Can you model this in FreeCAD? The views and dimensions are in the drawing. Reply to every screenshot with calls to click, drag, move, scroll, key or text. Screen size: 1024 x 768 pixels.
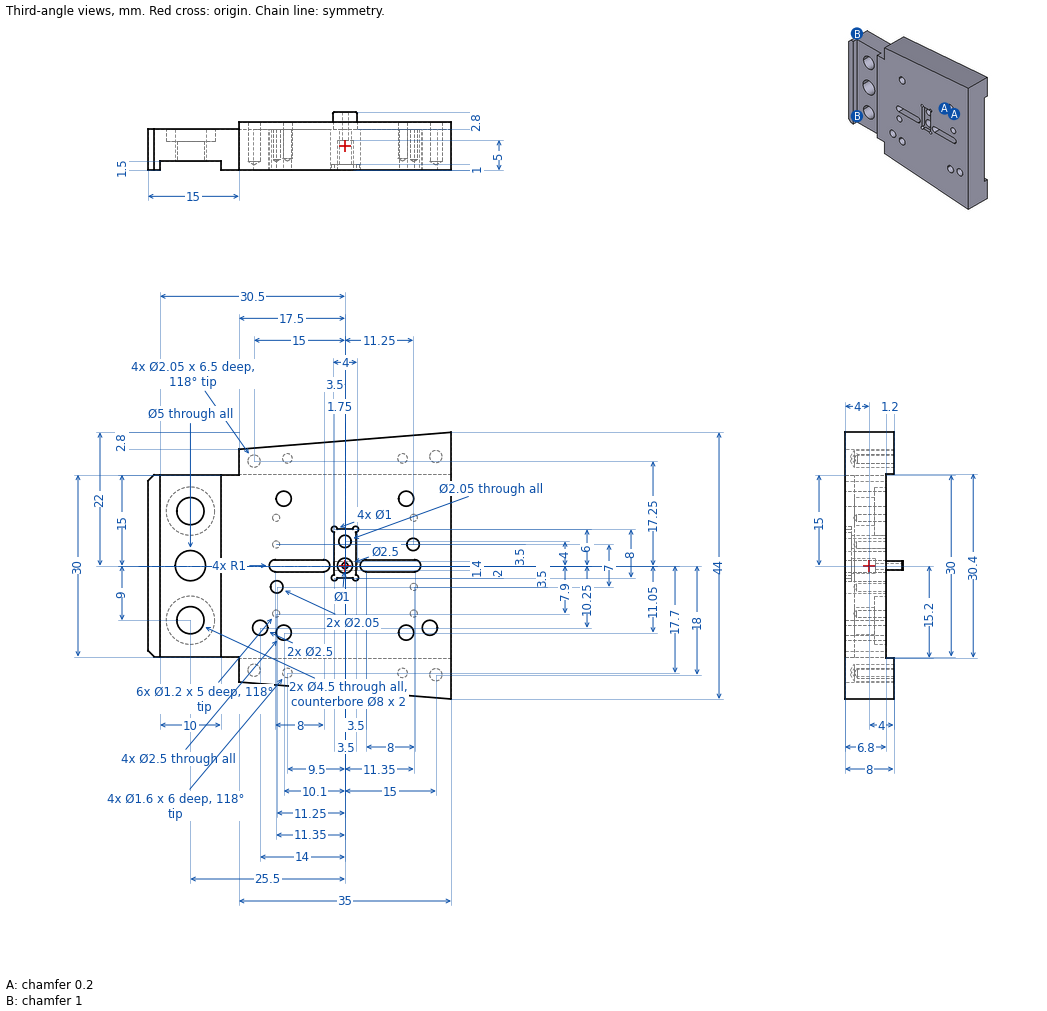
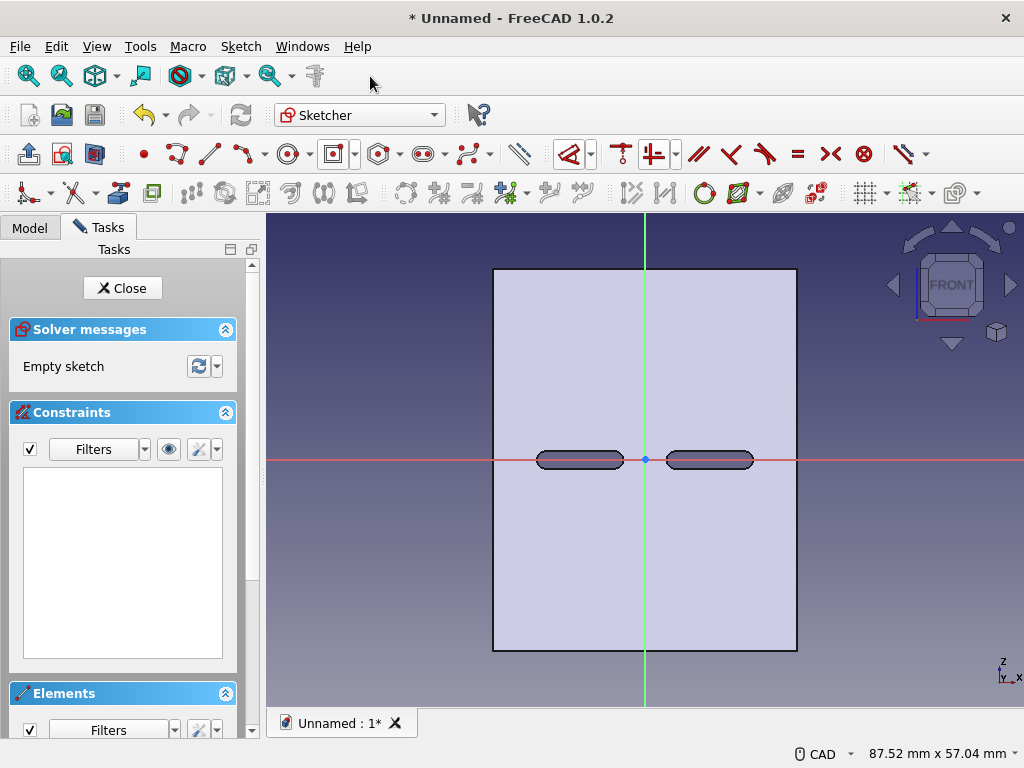
scroll(649, 460, up, 15)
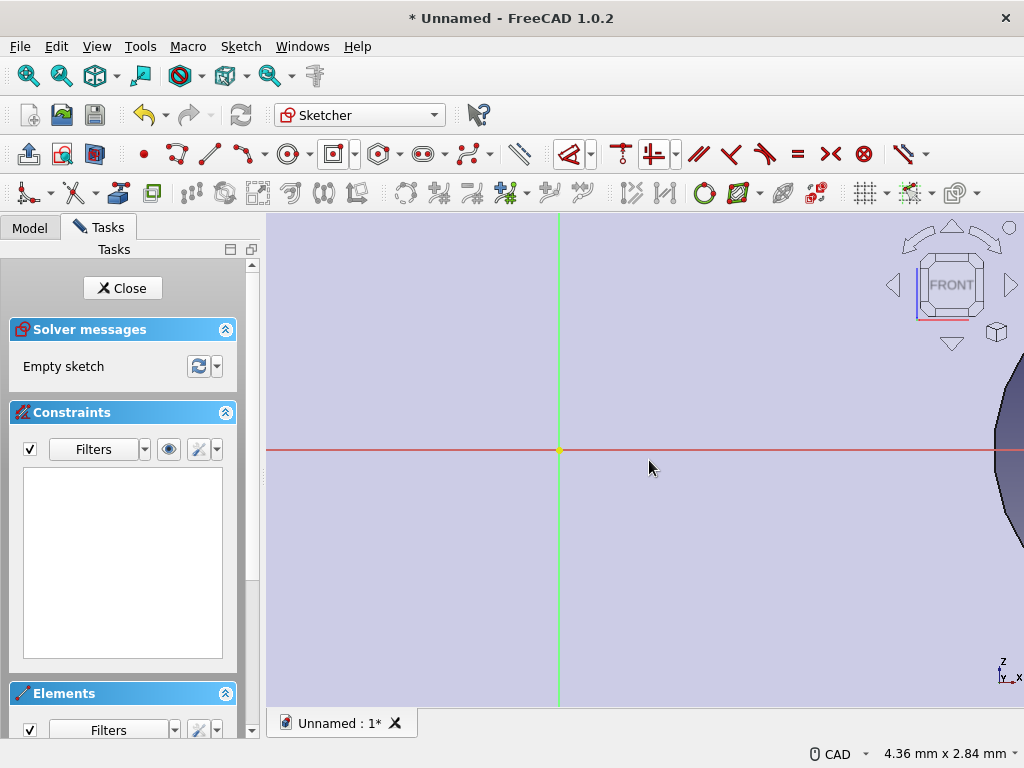
scroll(538, 439, up, 3)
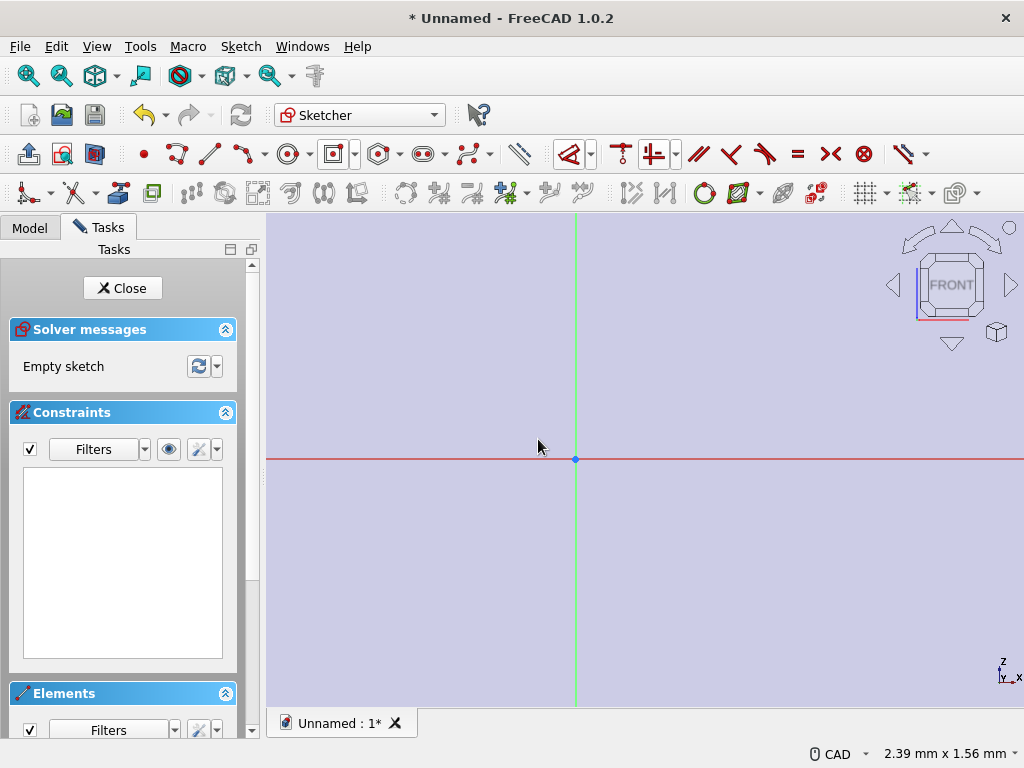
click(288, 154)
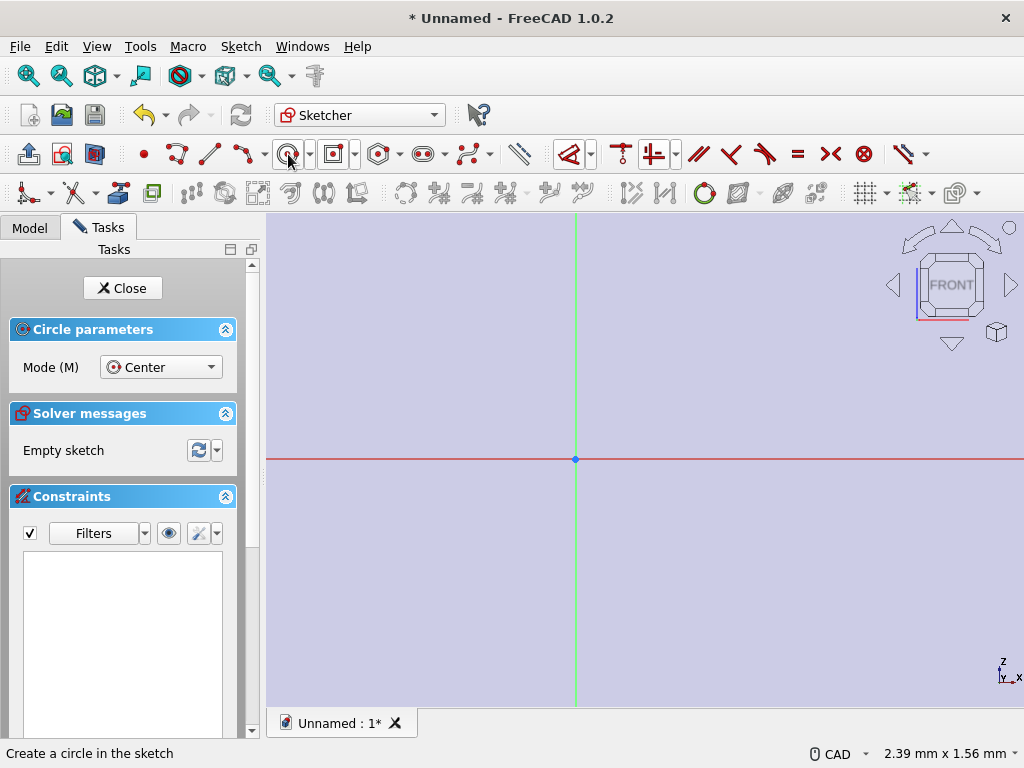
click(576, 459)
move(688, 347)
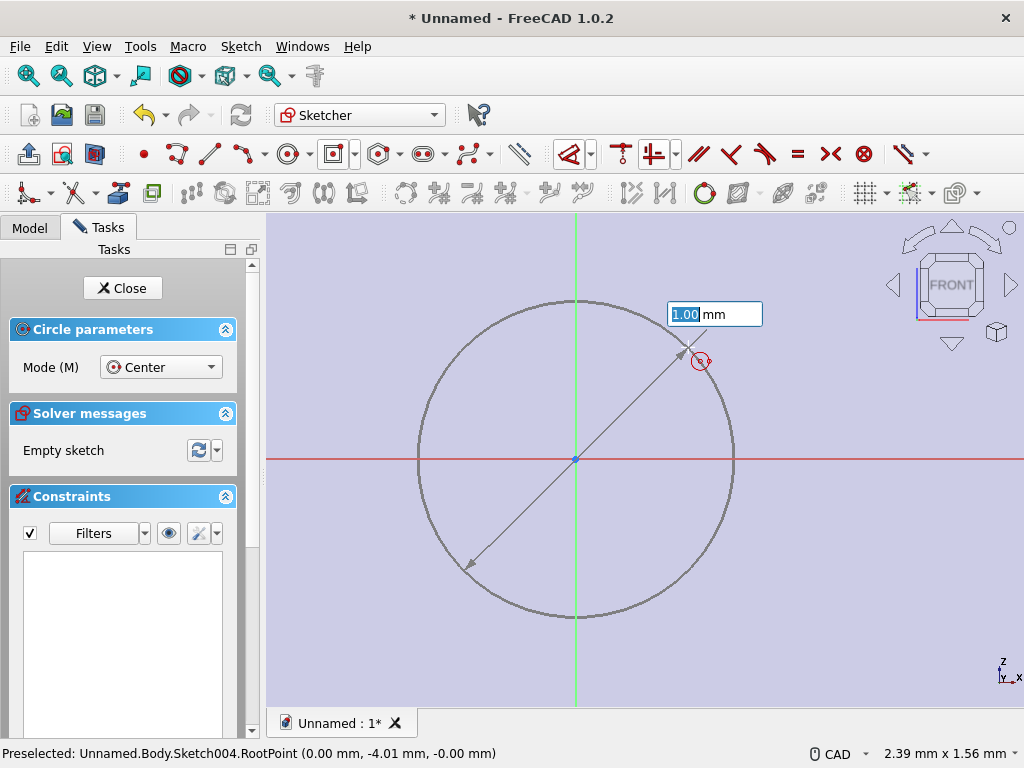
text(1)
key(Return)
key(Escape)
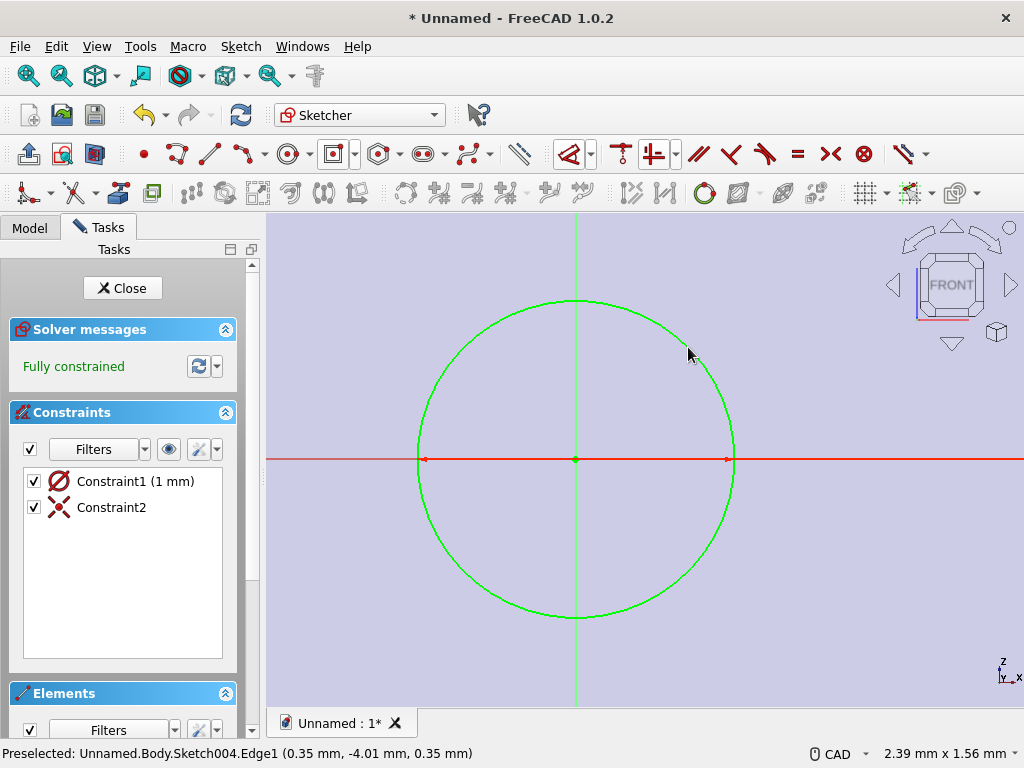
click(123, 288)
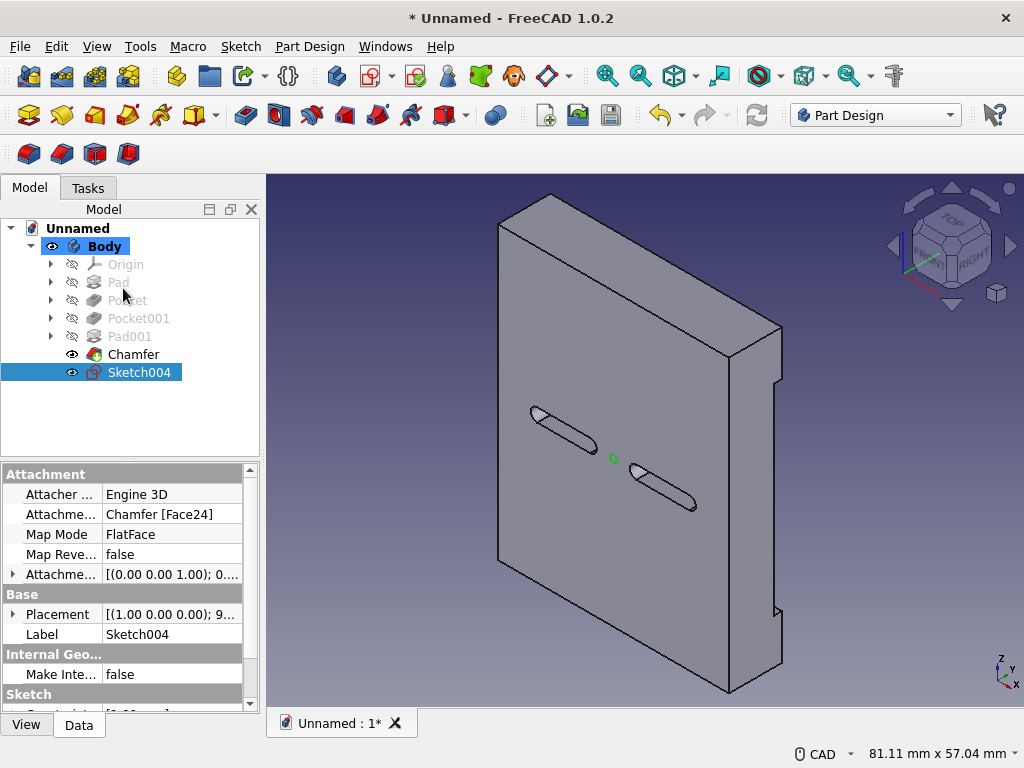
click(246, 116)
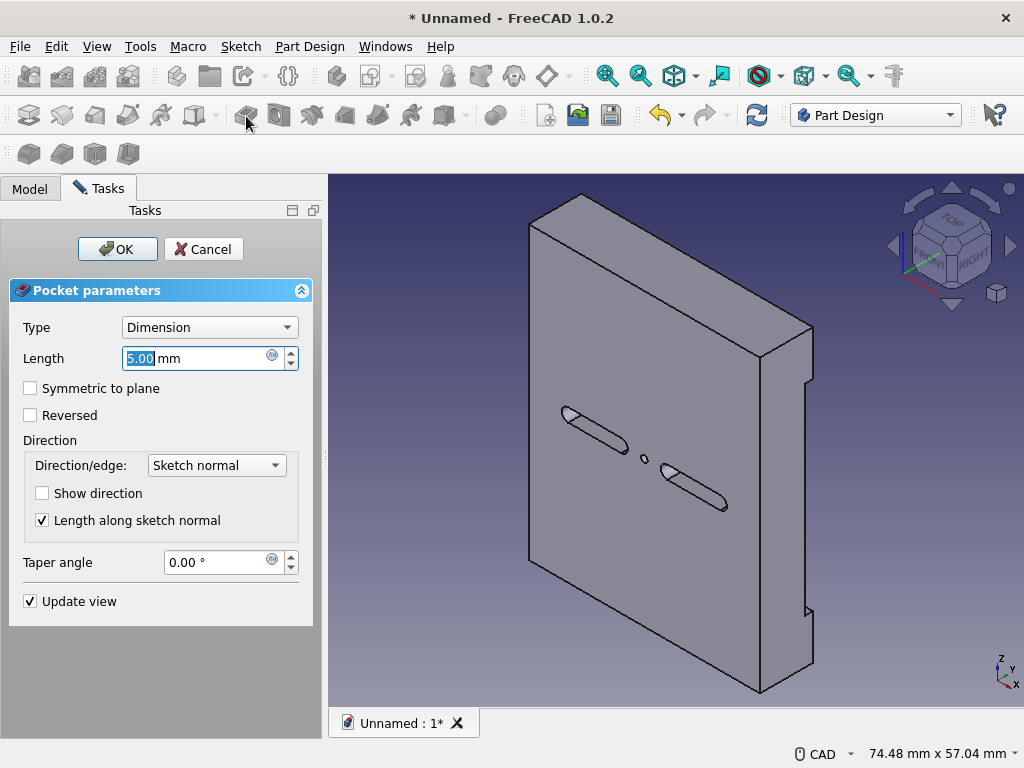
click(210, 328)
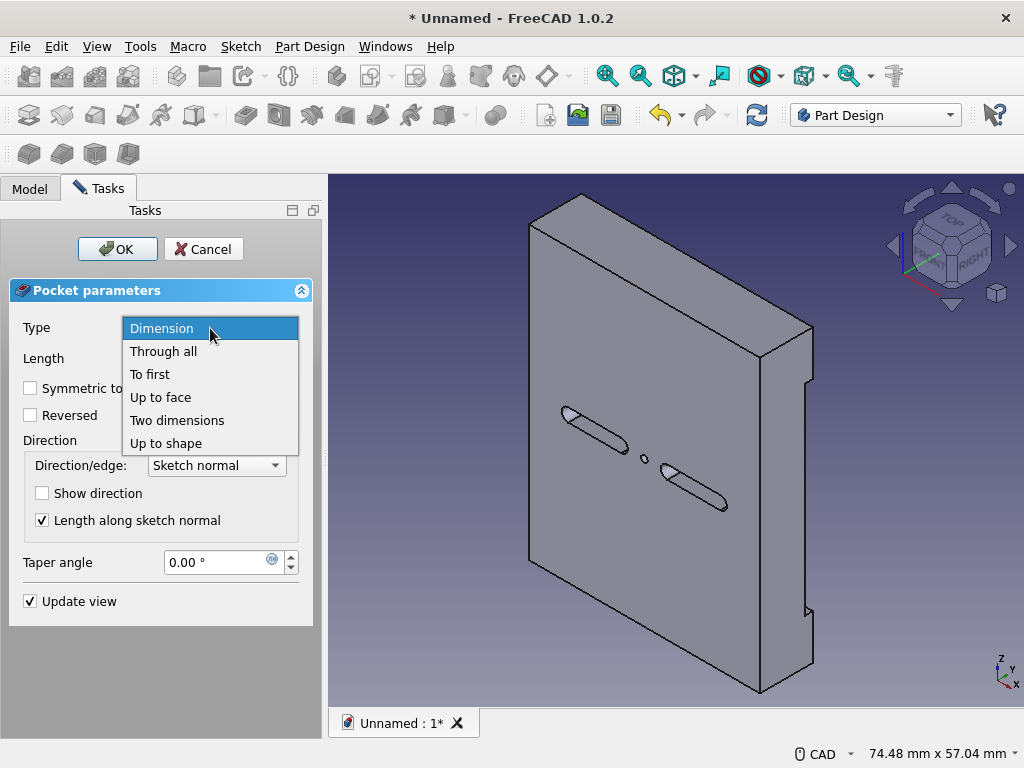
click(208, 352)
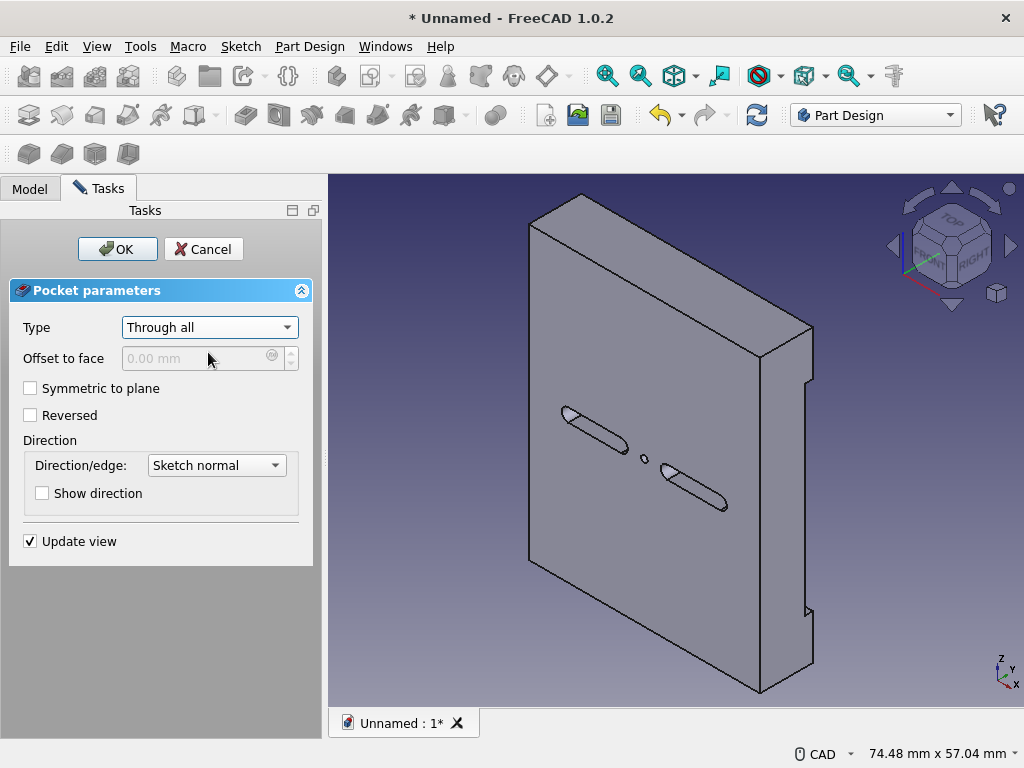
click(118, 249)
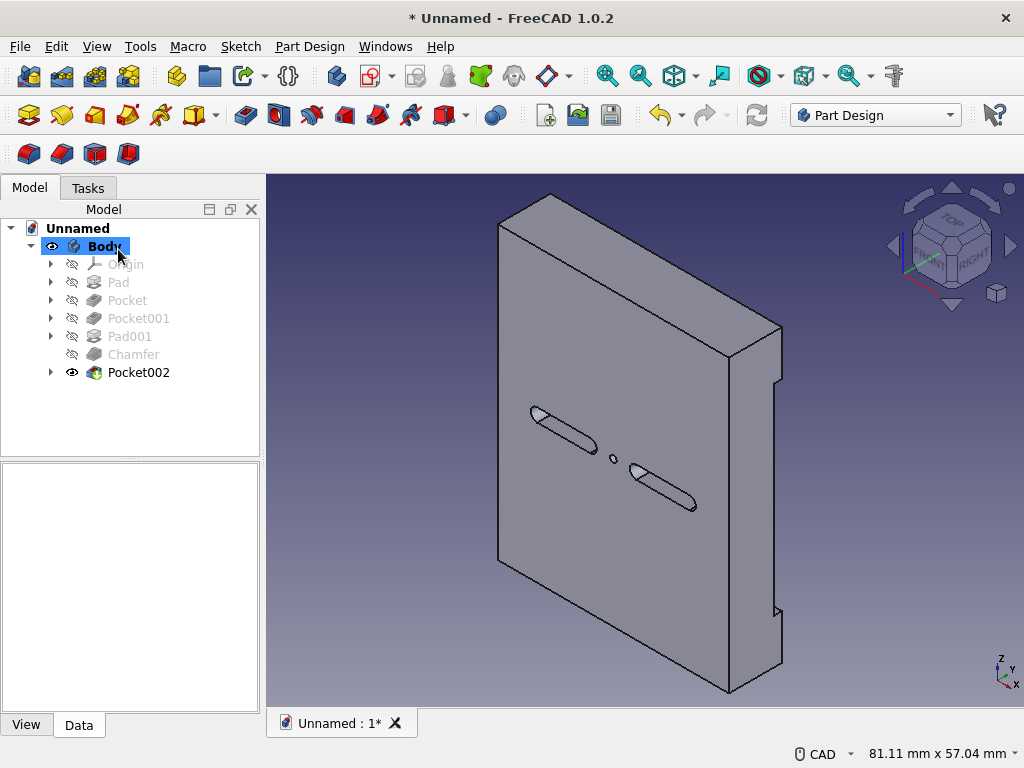
click(646, 573)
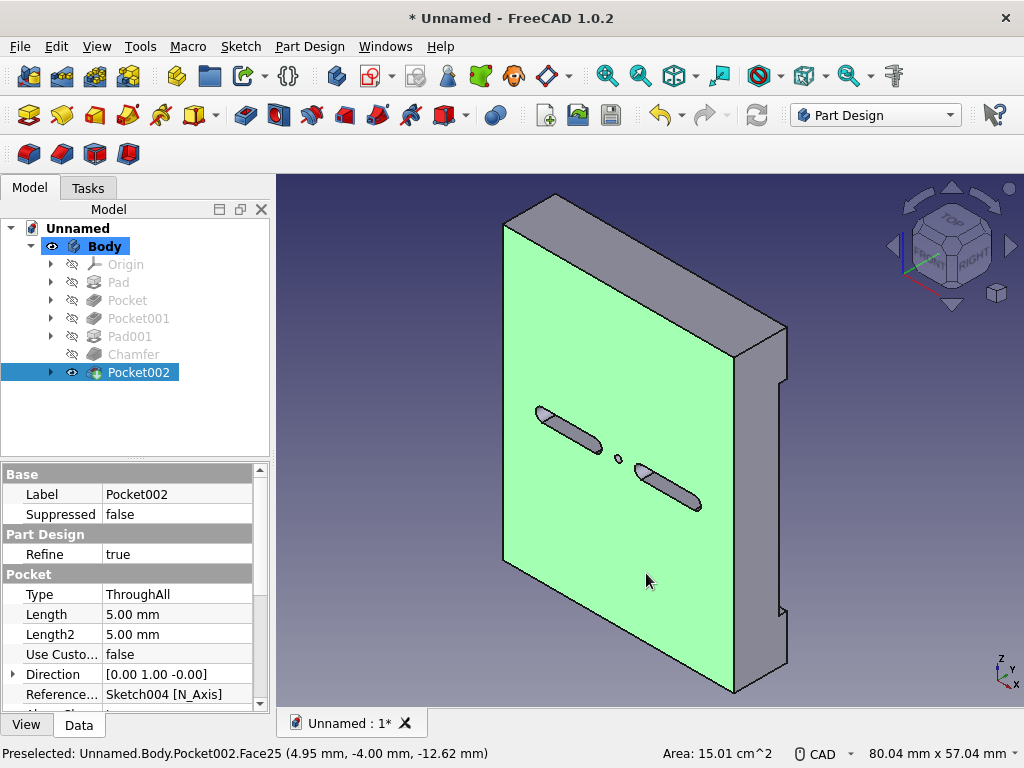
click(370, 76)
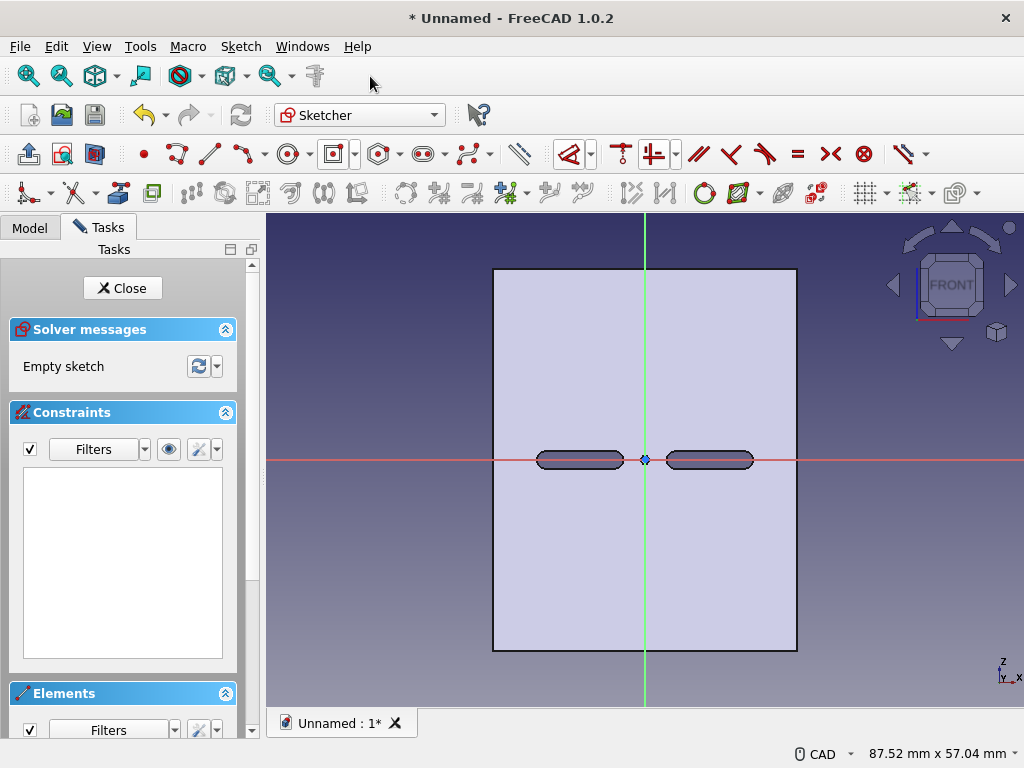
scroll(650, 460, up, 13)